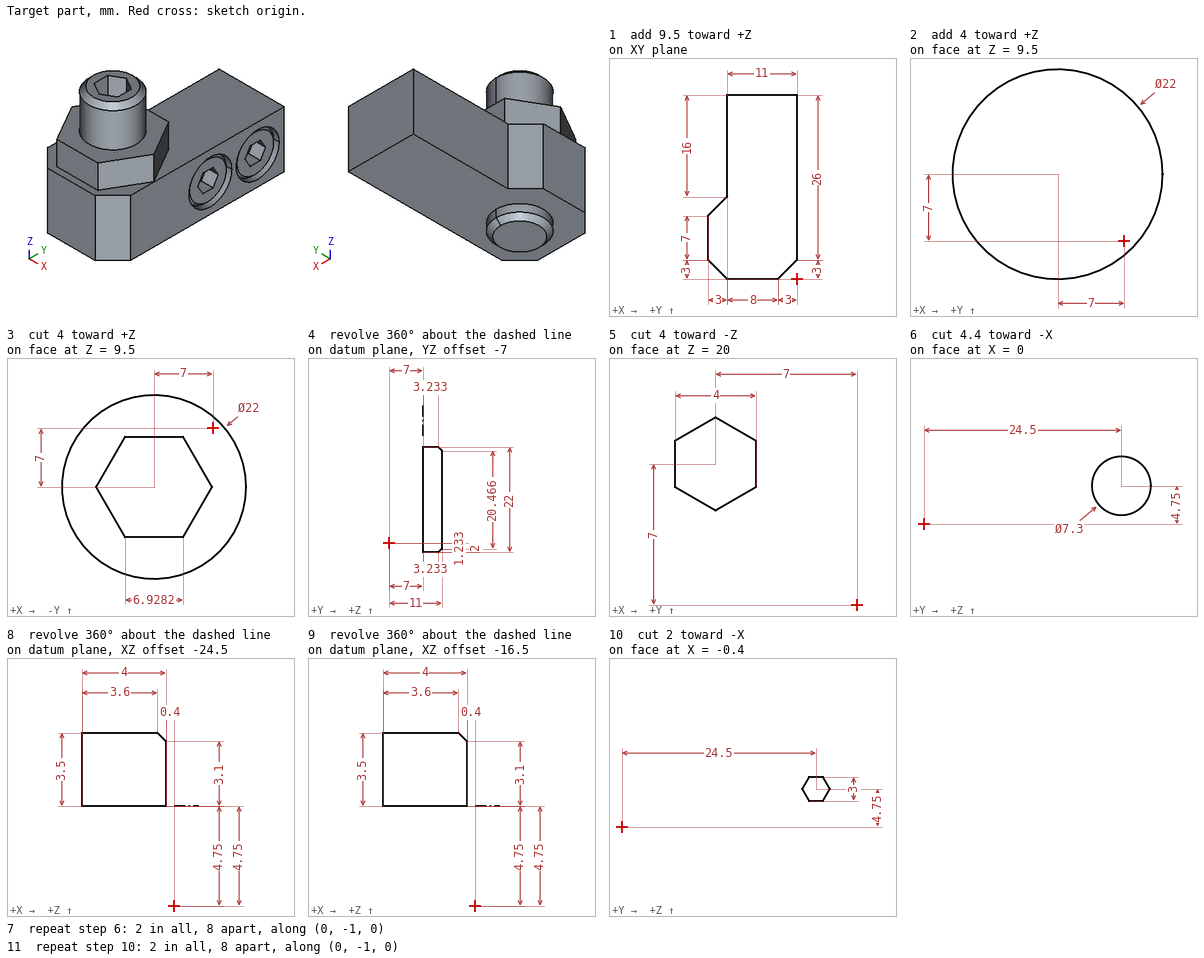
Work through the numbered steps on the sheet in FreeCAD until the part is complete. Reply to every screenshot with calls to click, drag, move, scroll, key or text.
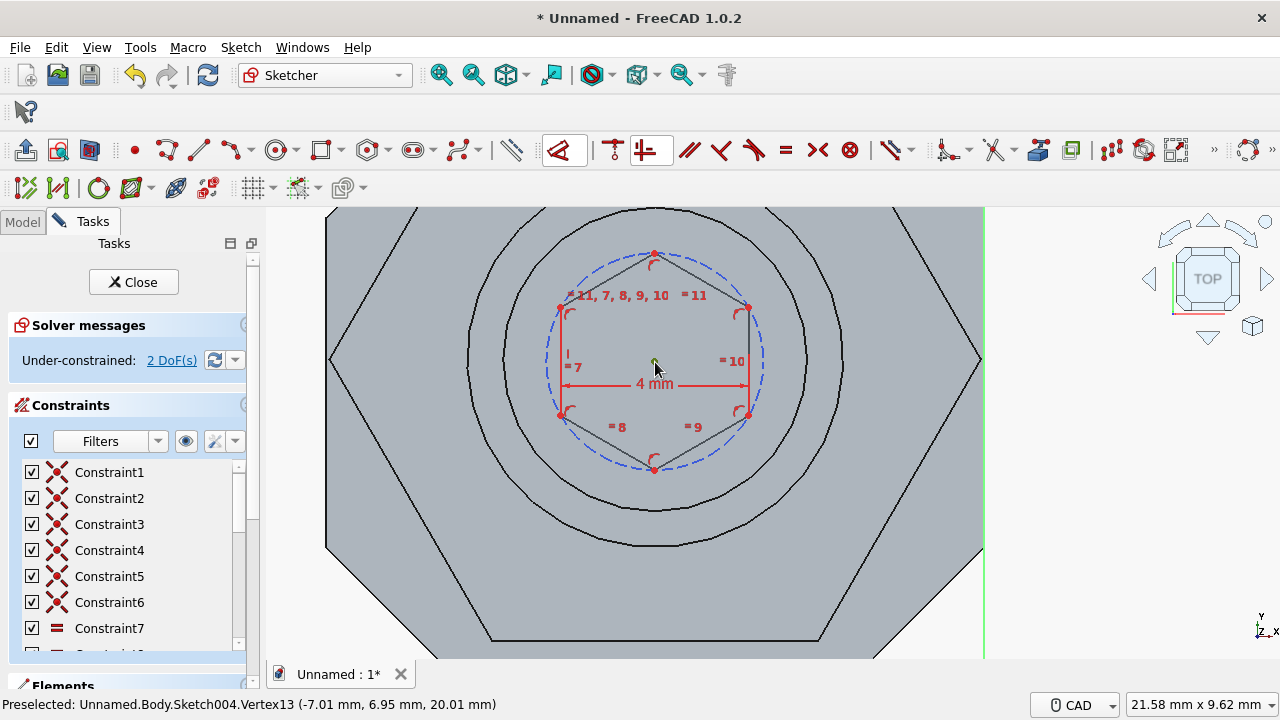
key(l)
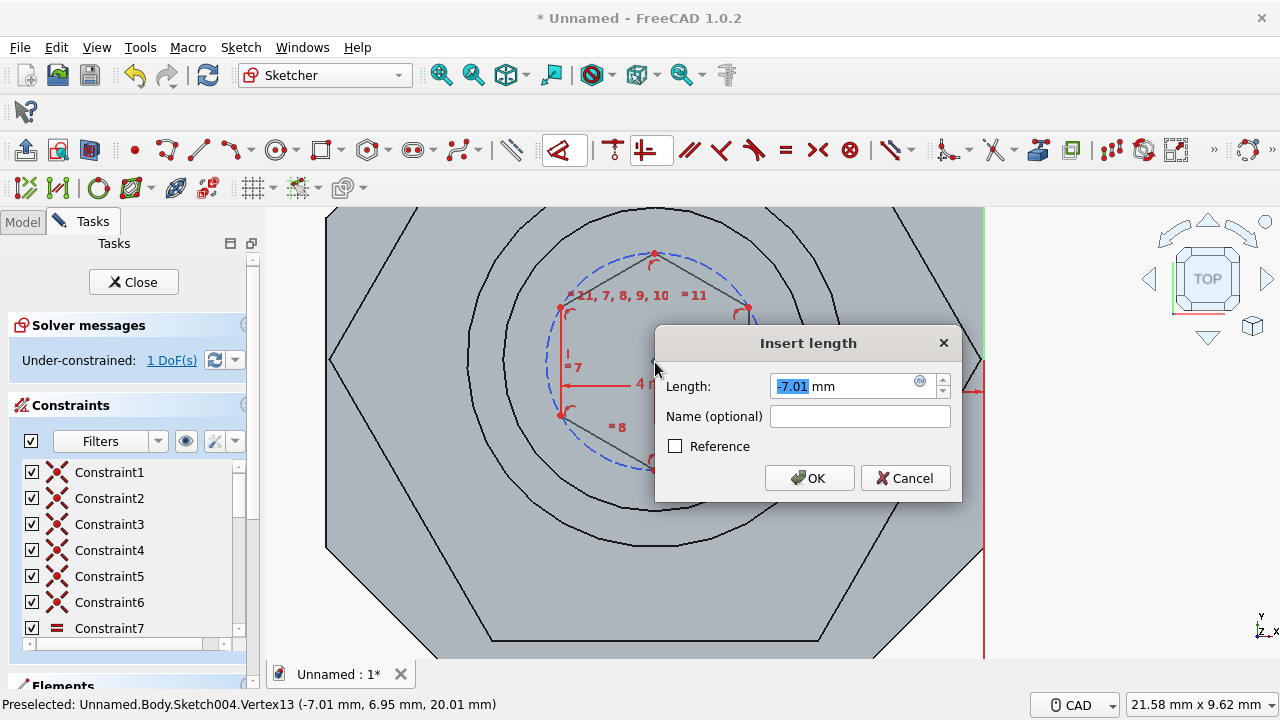
text(-7)
key(Return)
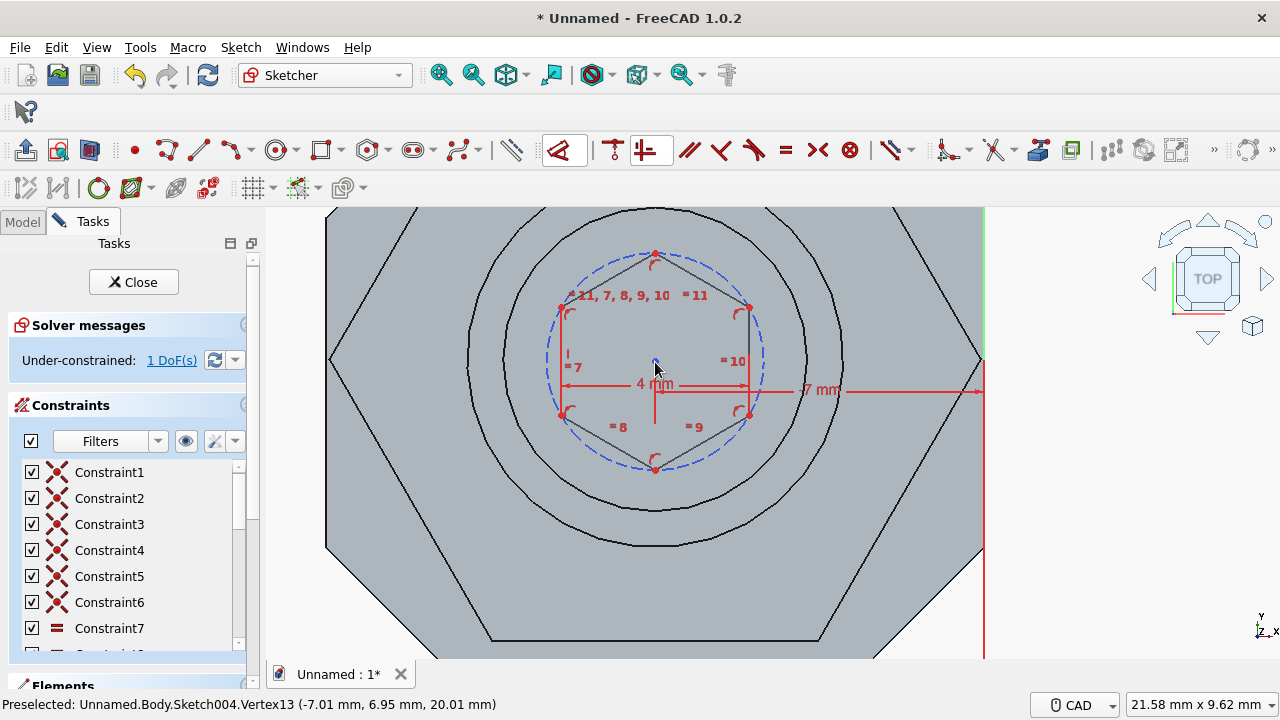
click(655, 362)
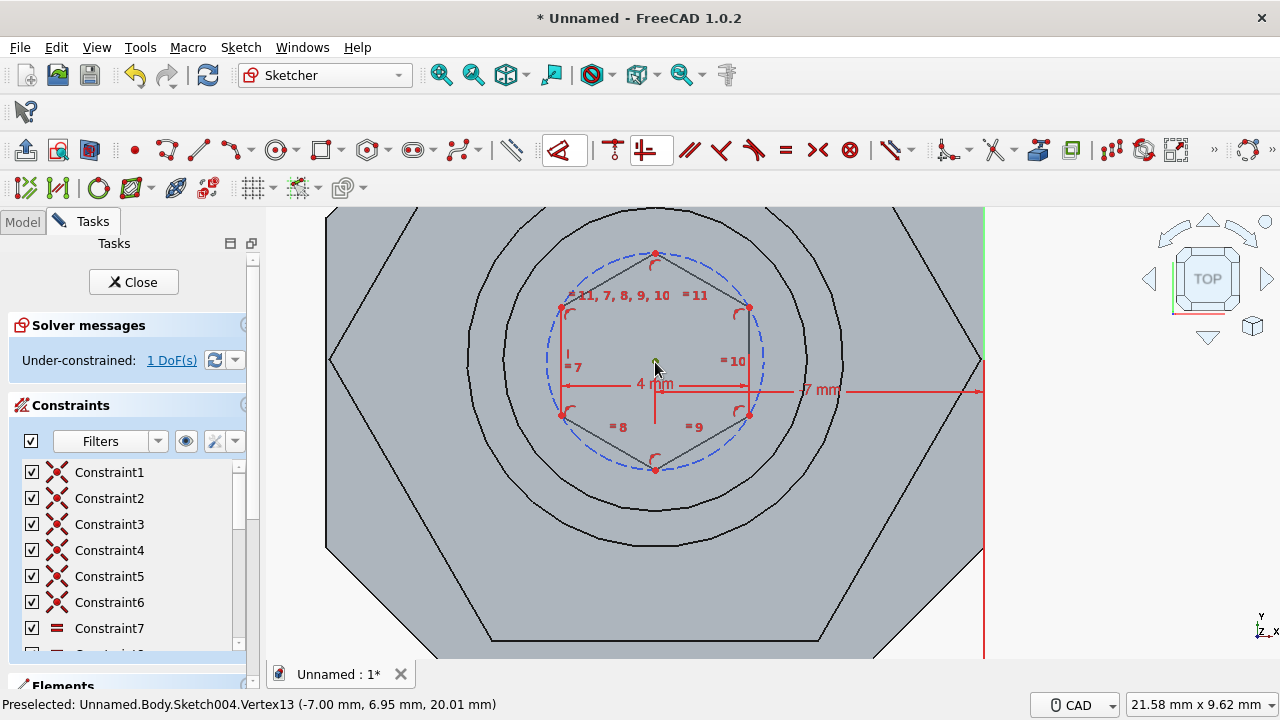
key(i)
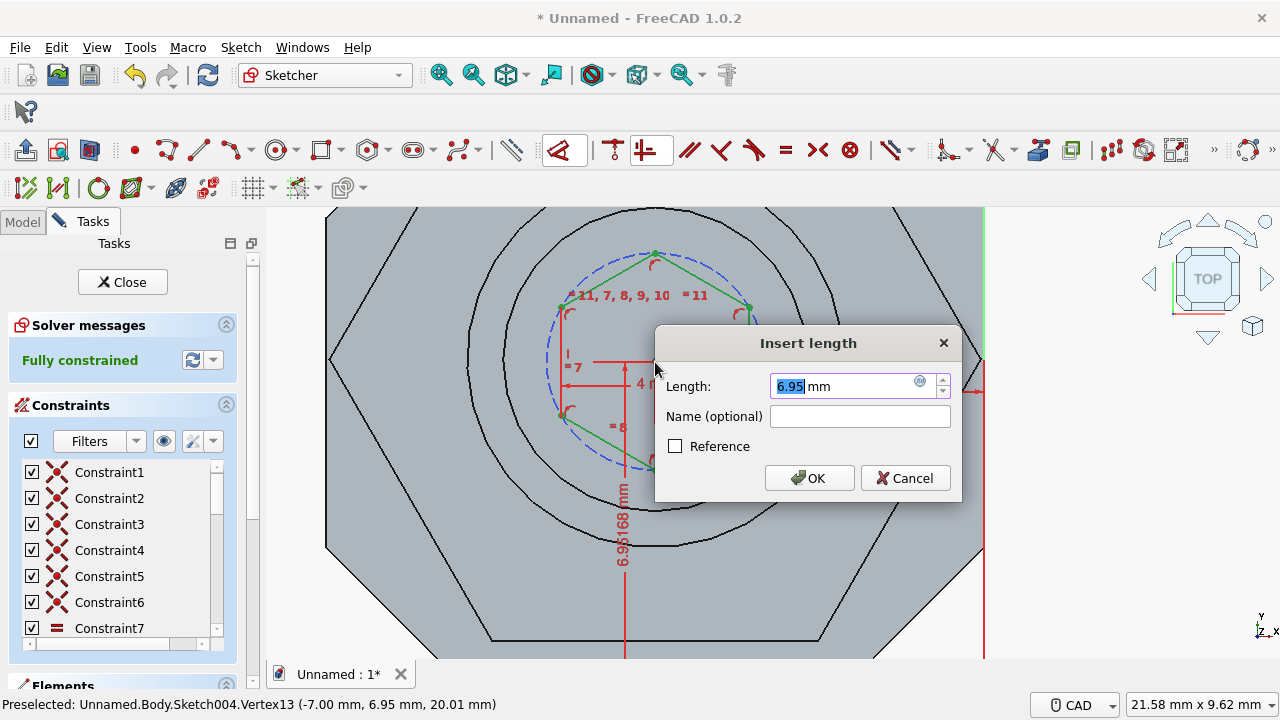
text(7)
key(Return)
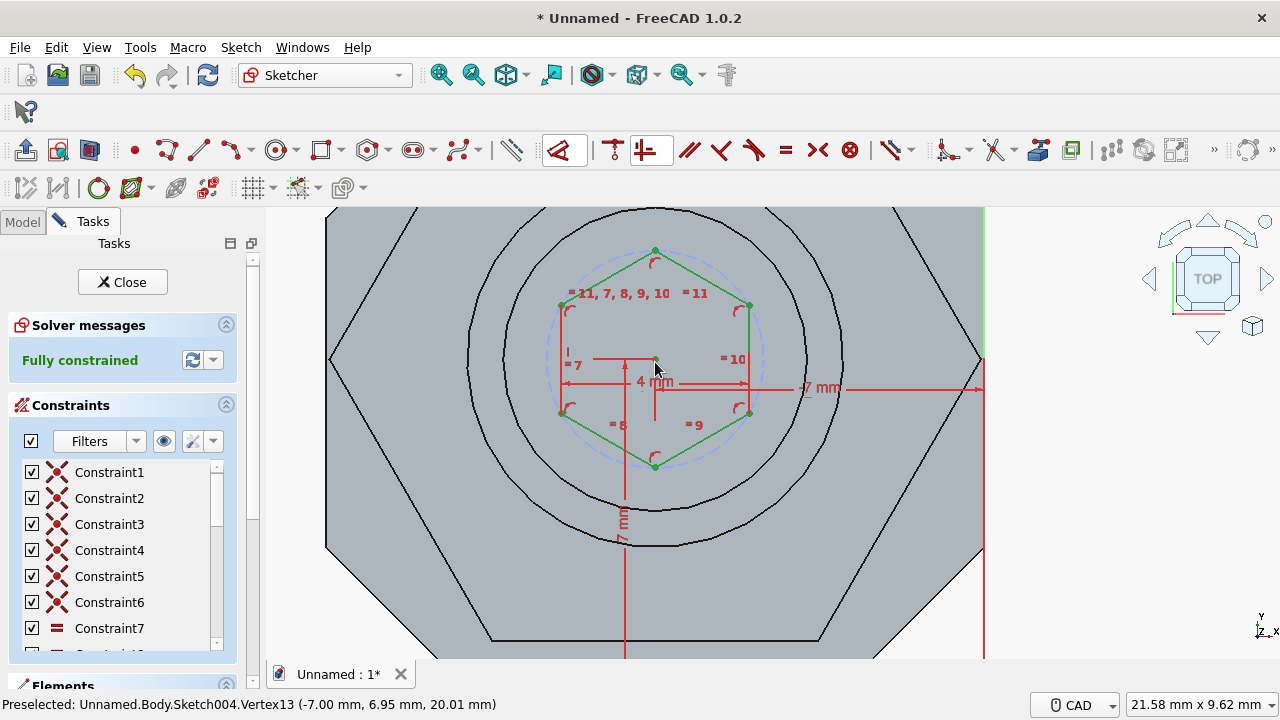
click(123, 282)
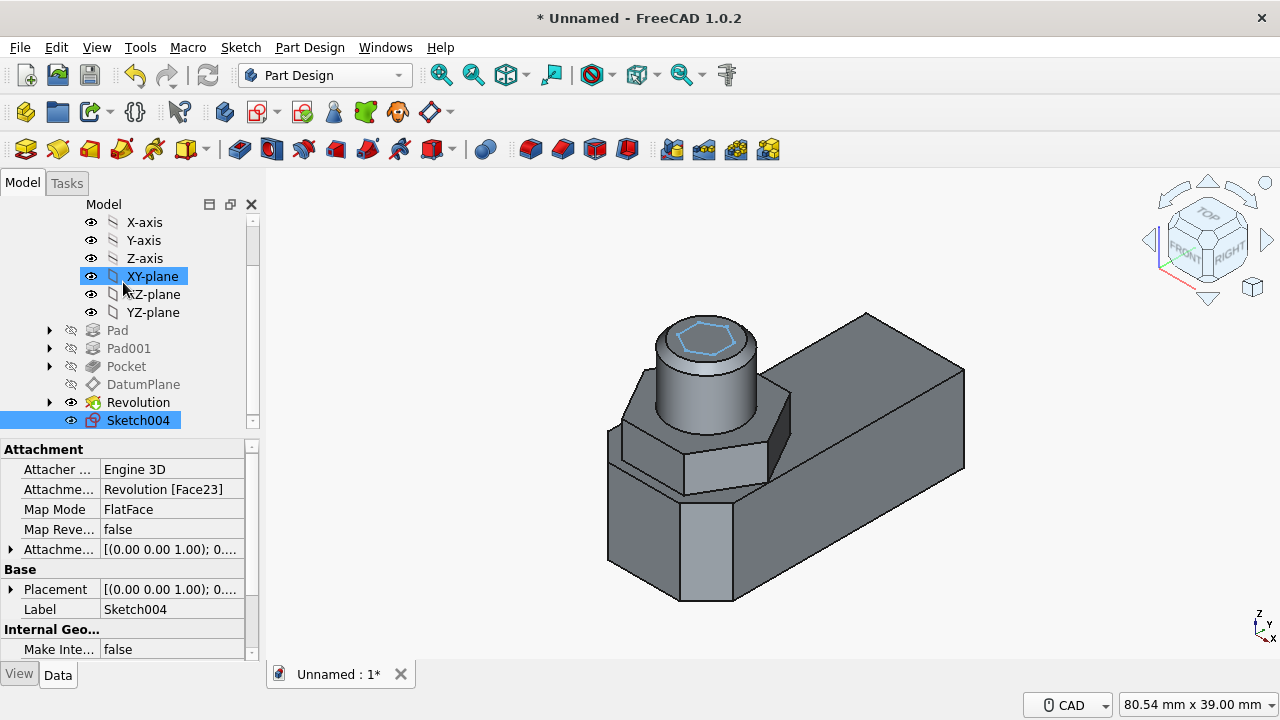
click(240, 150)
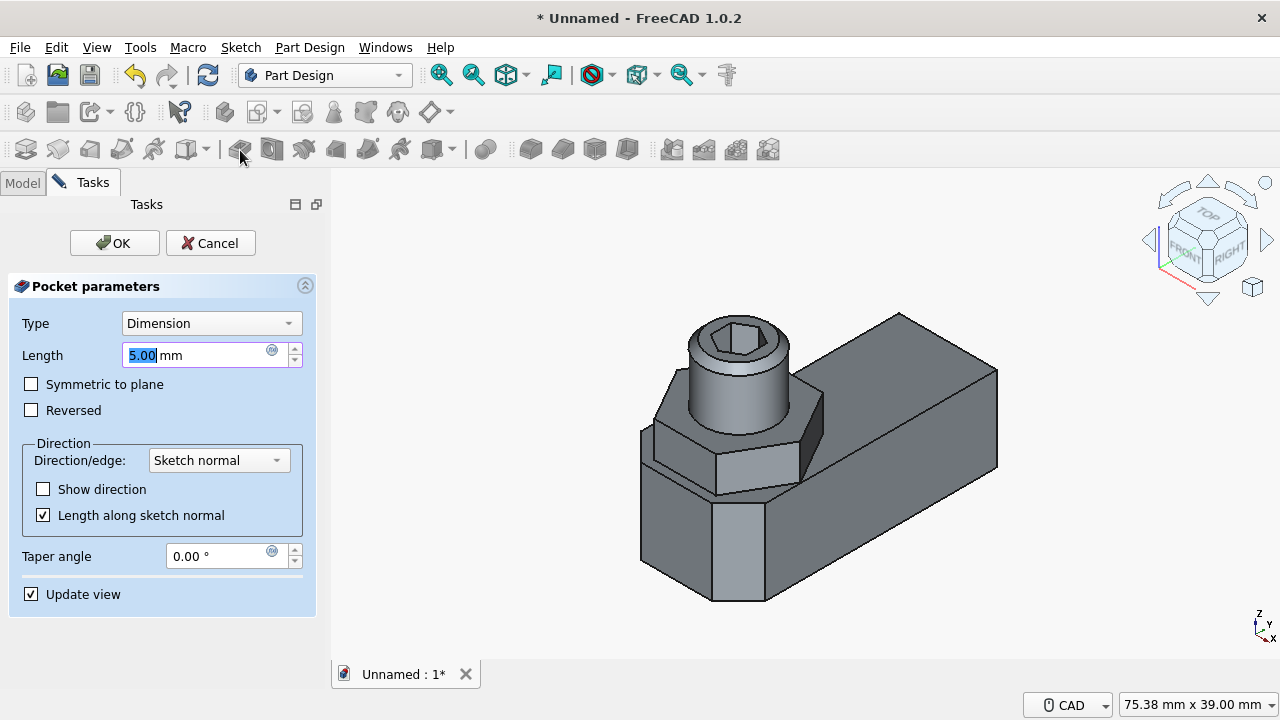
text(4)
key(Tab)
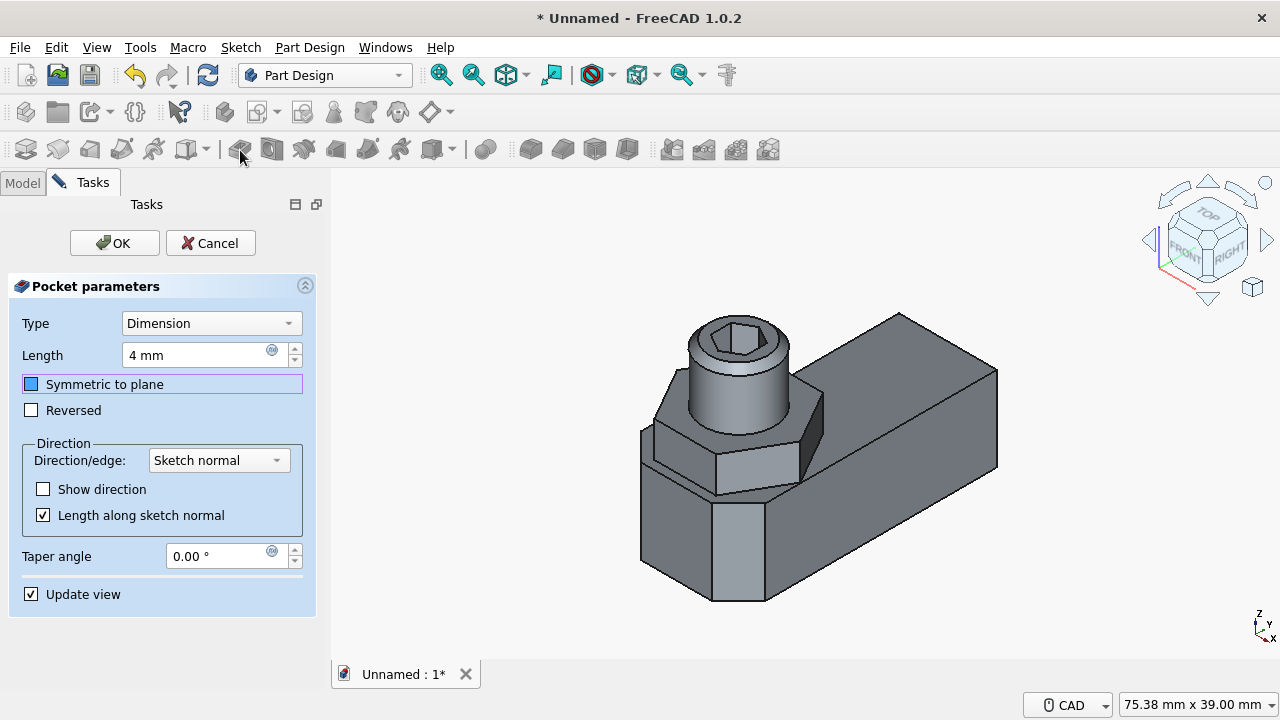
click(115, 243)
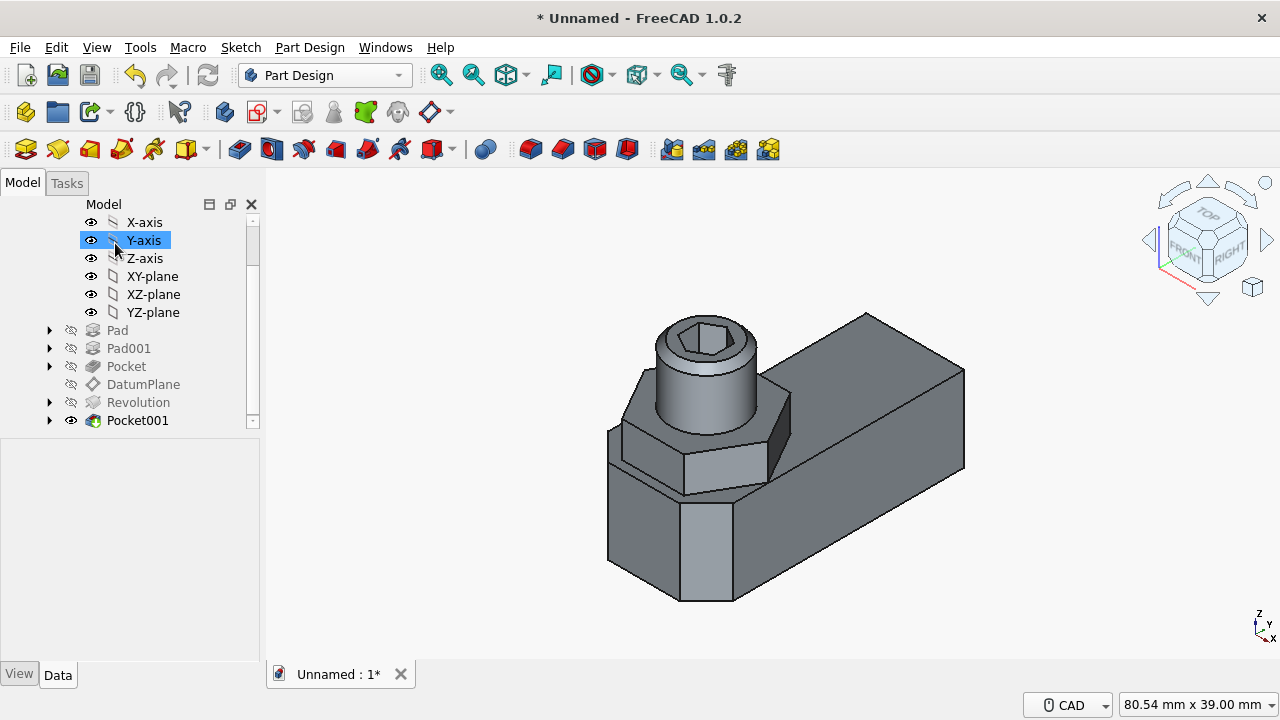
click(915, 446)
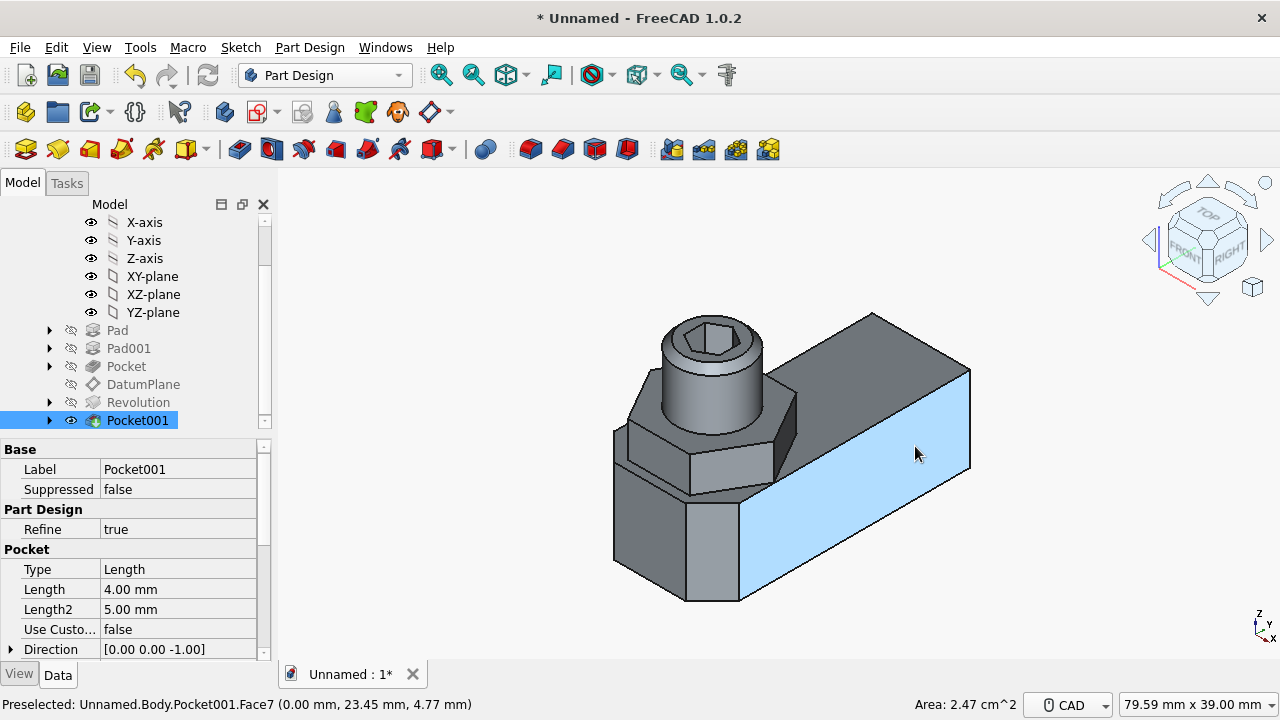
click(258, 112)